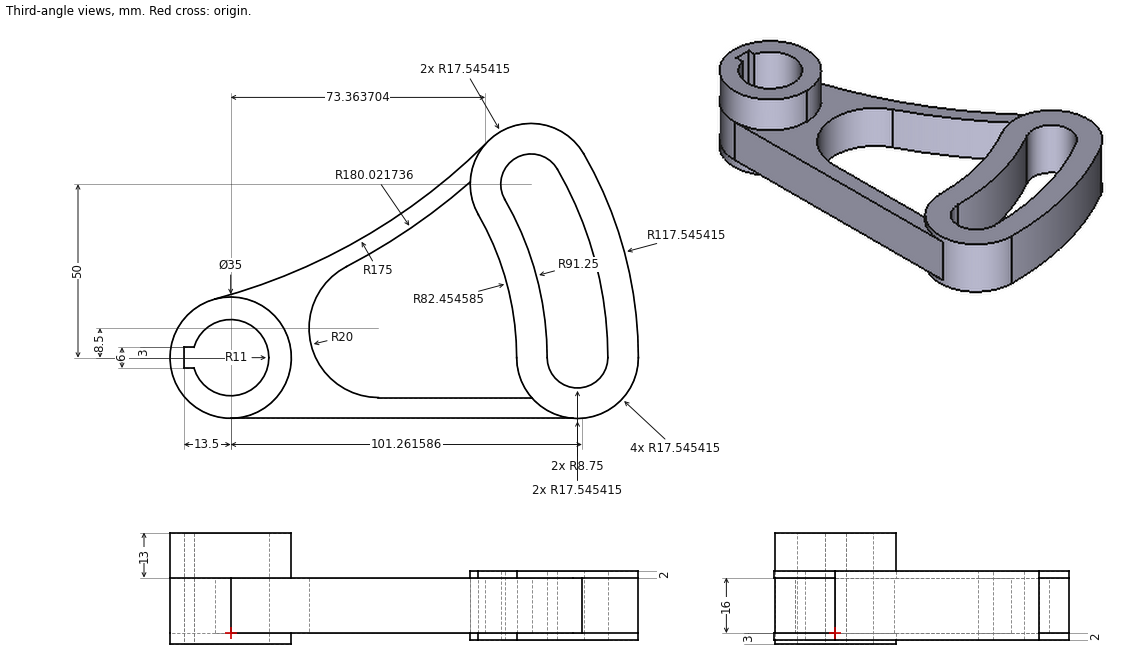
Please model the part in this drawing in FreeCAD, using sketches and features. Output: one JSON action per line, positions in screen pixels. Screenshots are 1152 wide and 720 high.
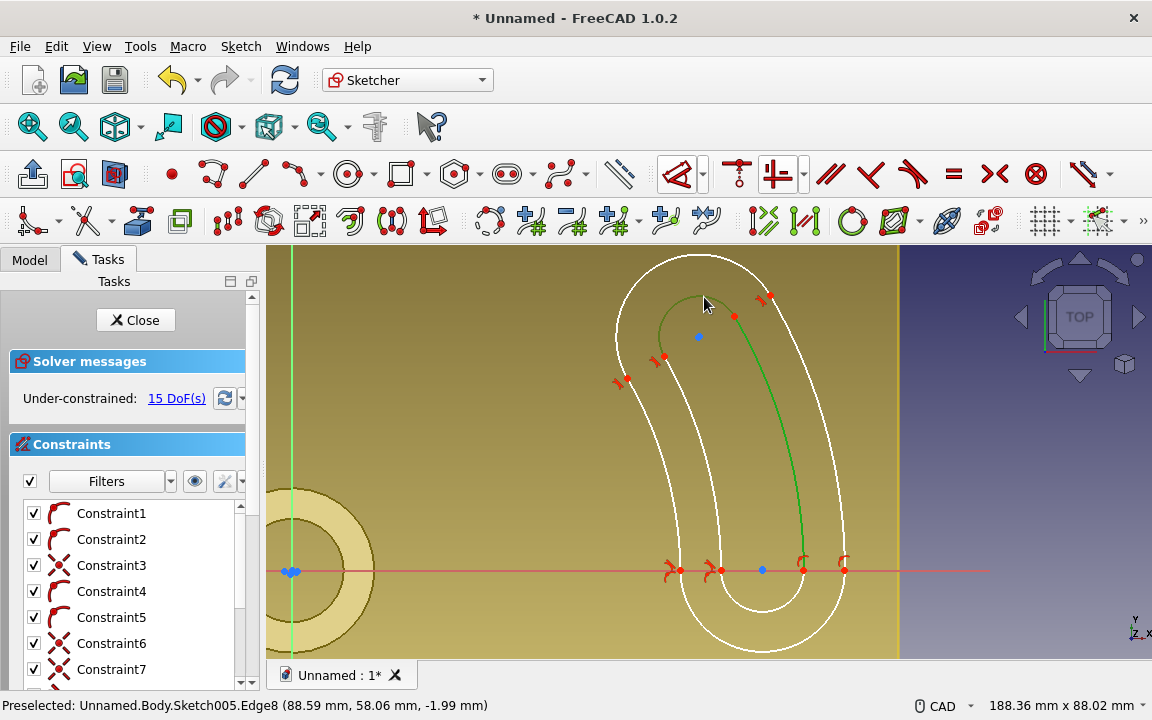
{"action": "left_click", "coordinate": [913, 174]}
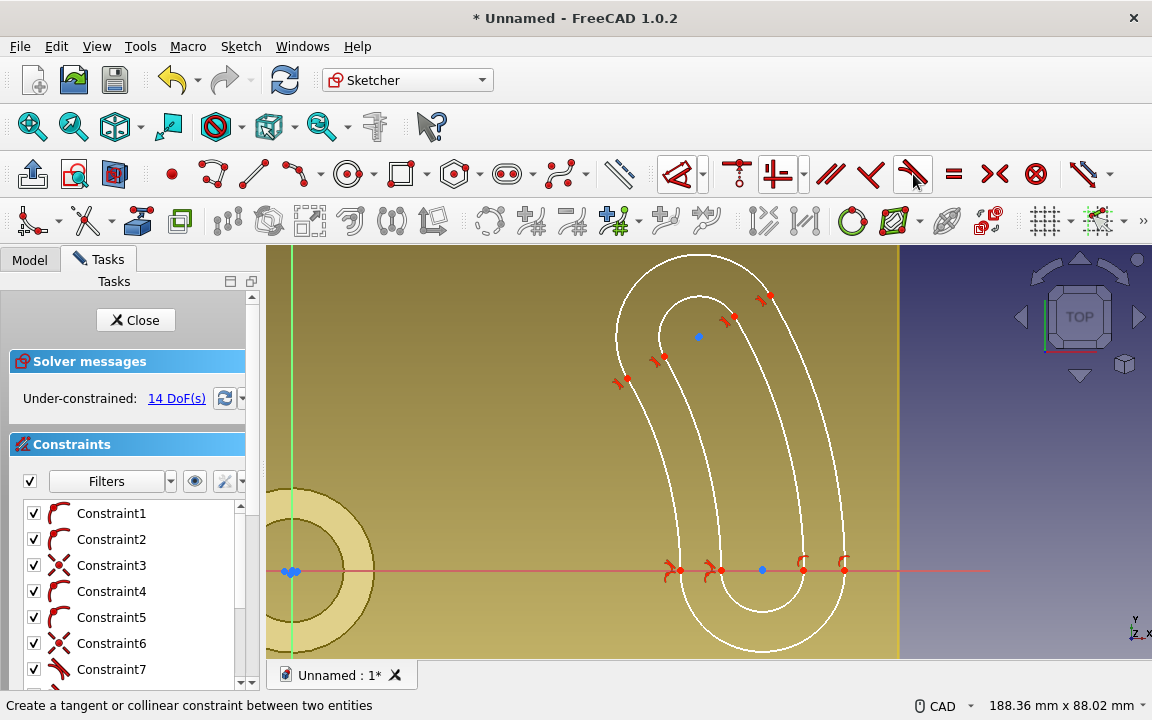
{"action": "left_click", "coordinate": [675, 510]}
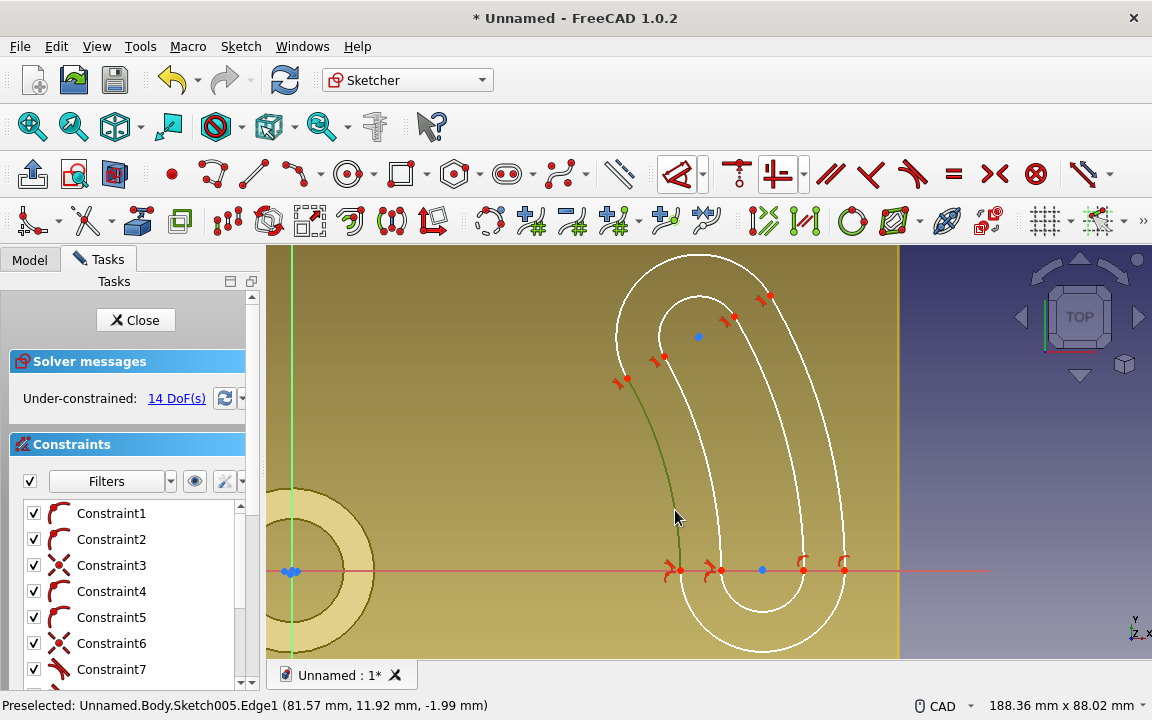
{"action": "left_click", "coordinate": [838, 484]}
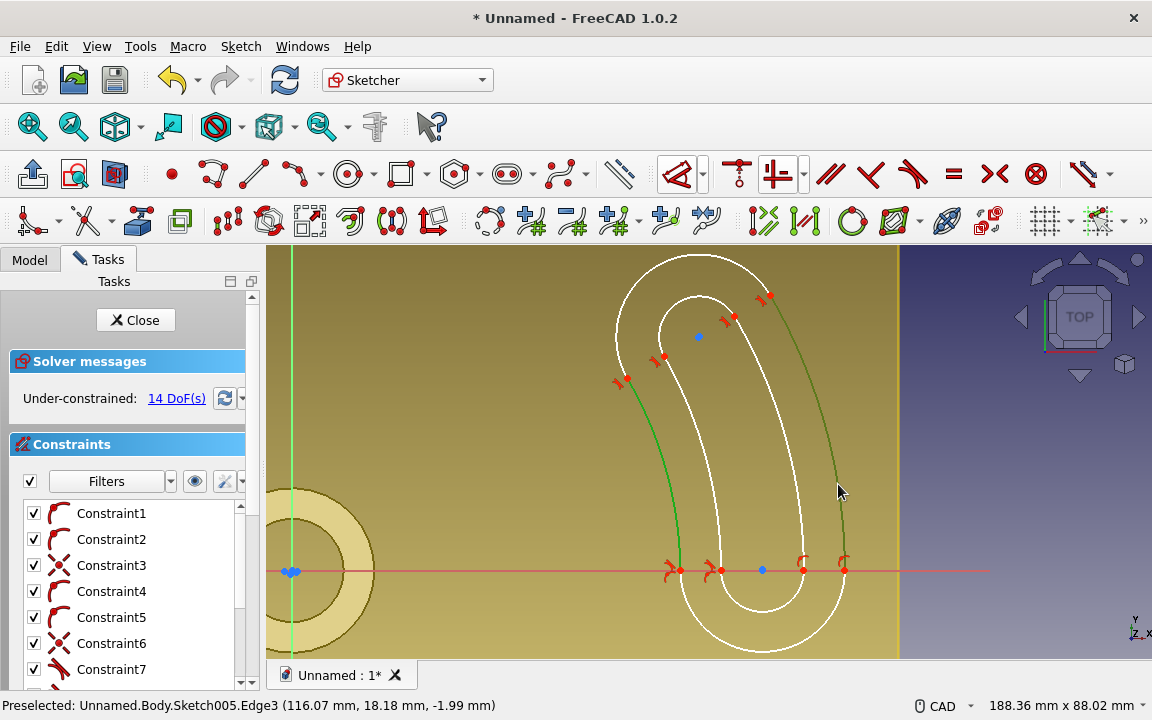
{"action": "left_click", "coordinate": [737, 174]}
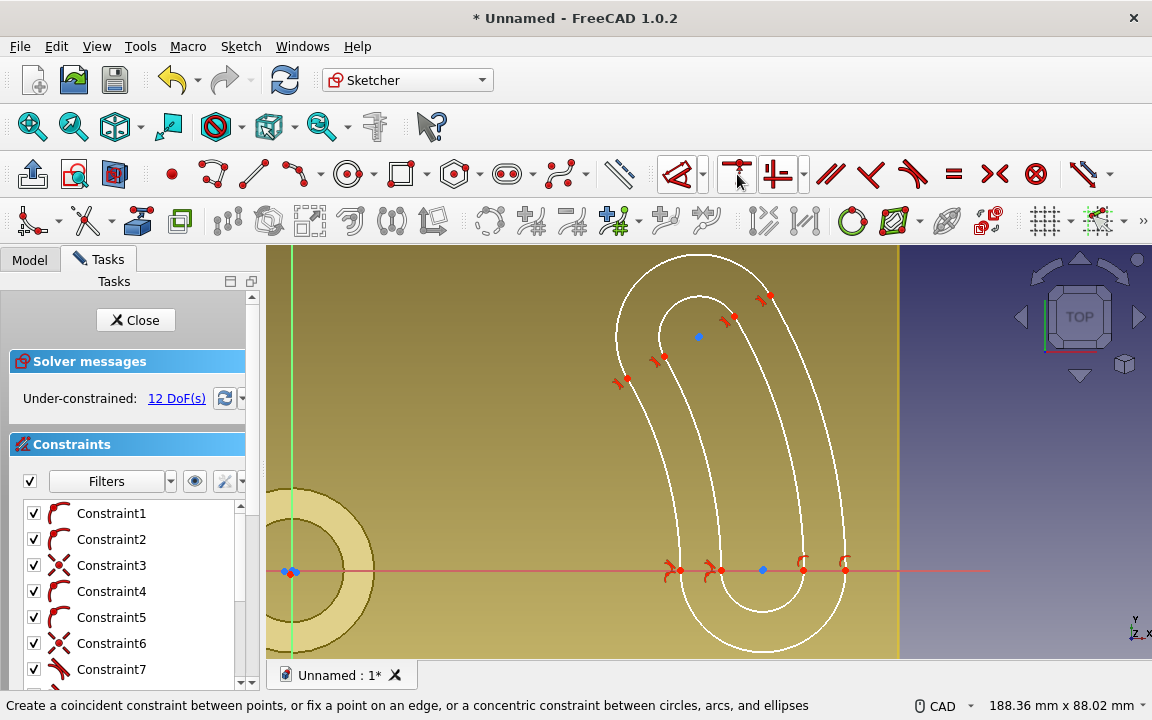
{"action": "left_click", "coordinate": [675, 510]}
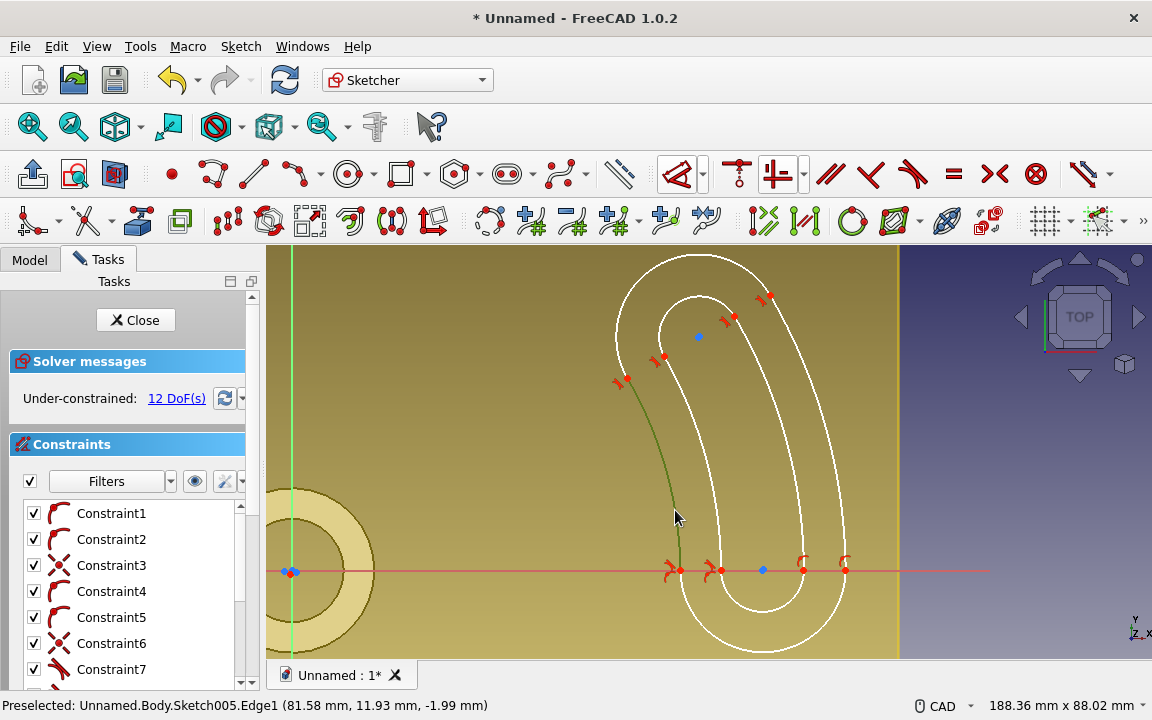
{"action": "left_click", "coordinate": [716, 504]}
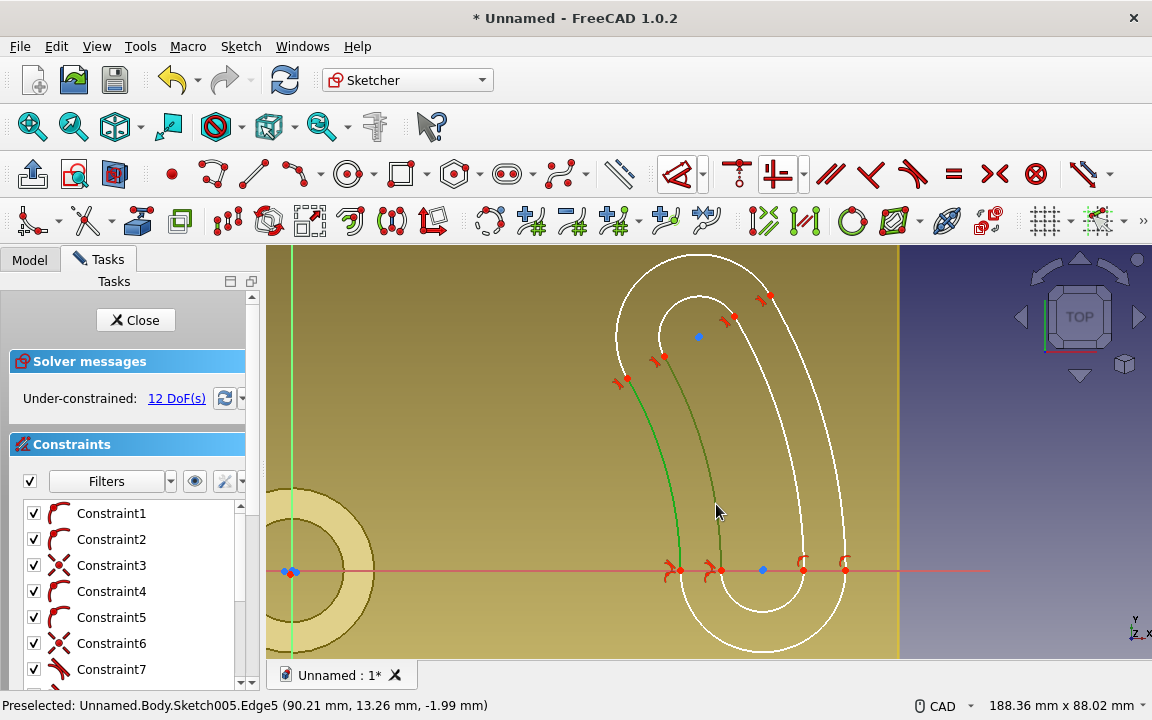
{"action": "left_click", "coordinate": [737, 174]}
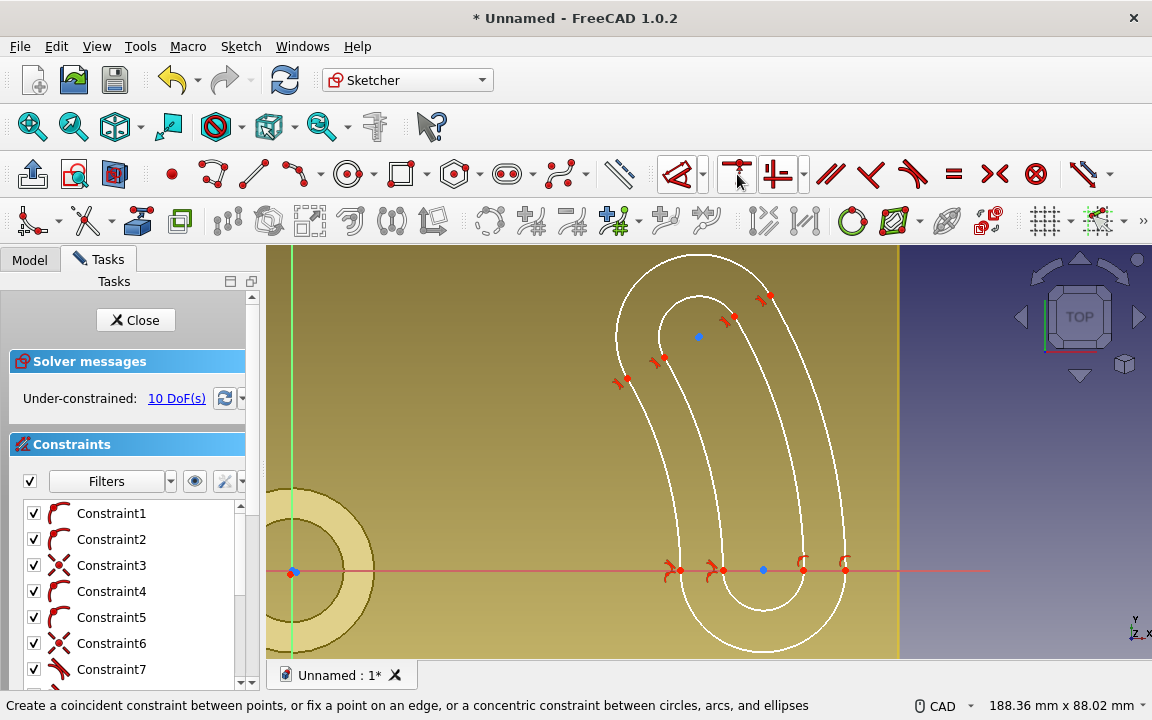
{"action": "left_click", "coordinate": [675, 510]}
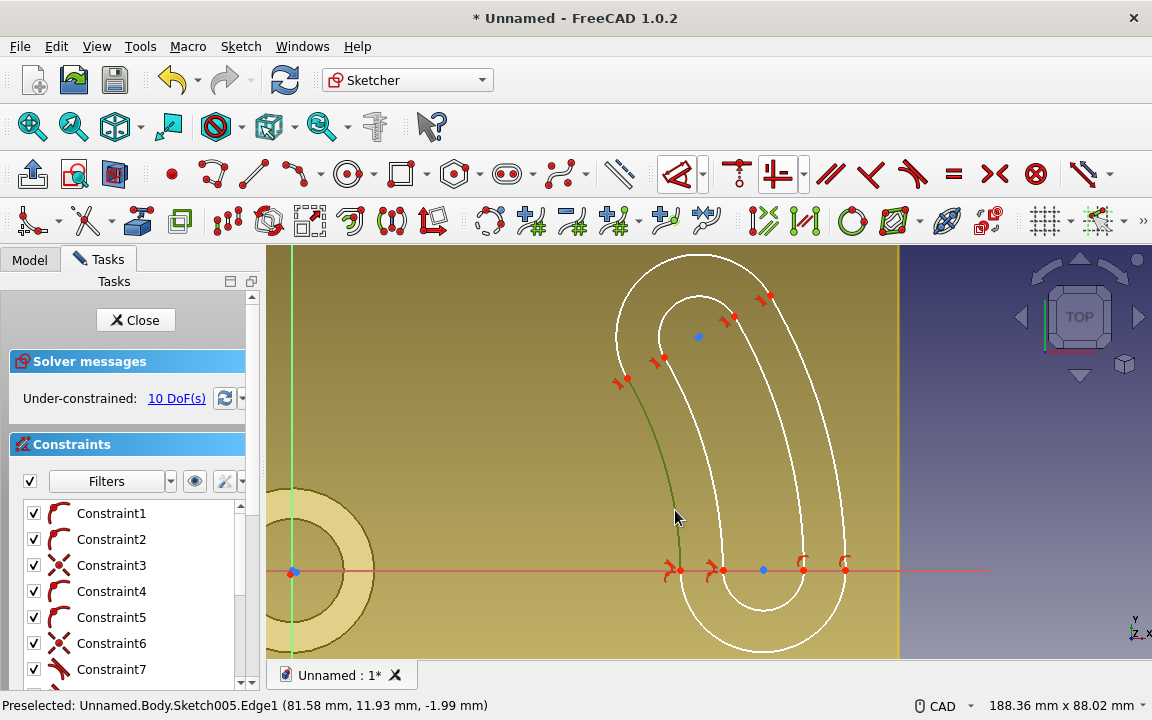
{"action": "left_click", "coordinate": [797, 491]}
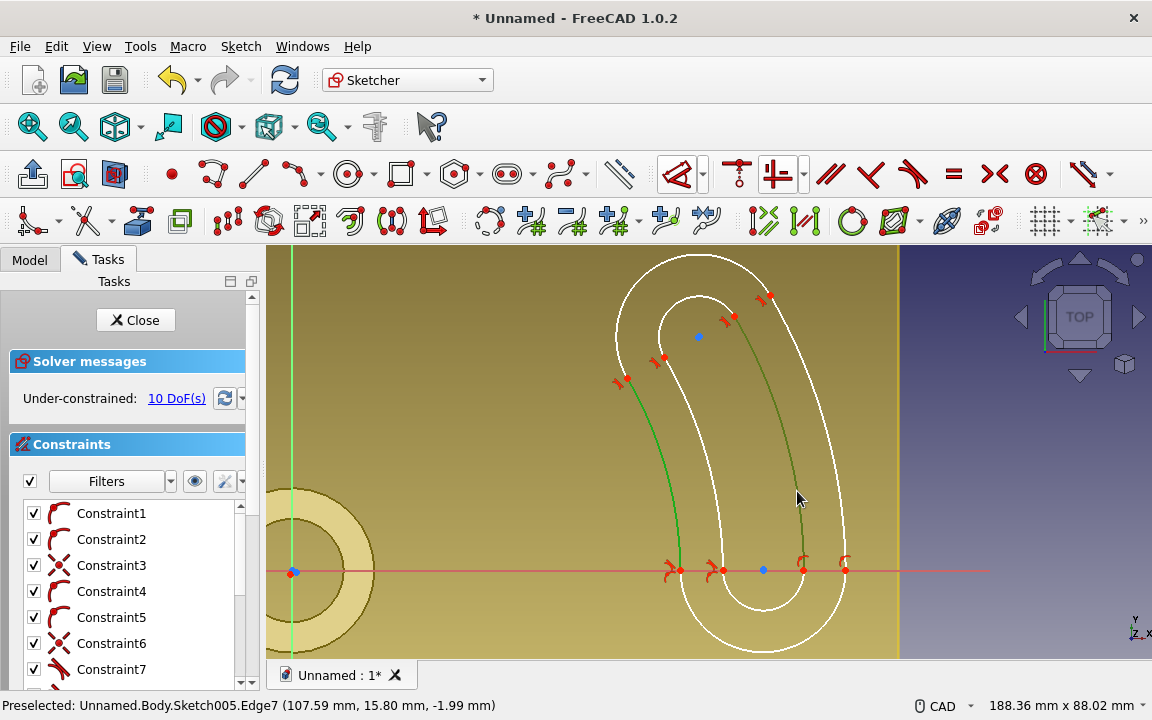
{"action": "left_click", "coordinate": [737, 174]}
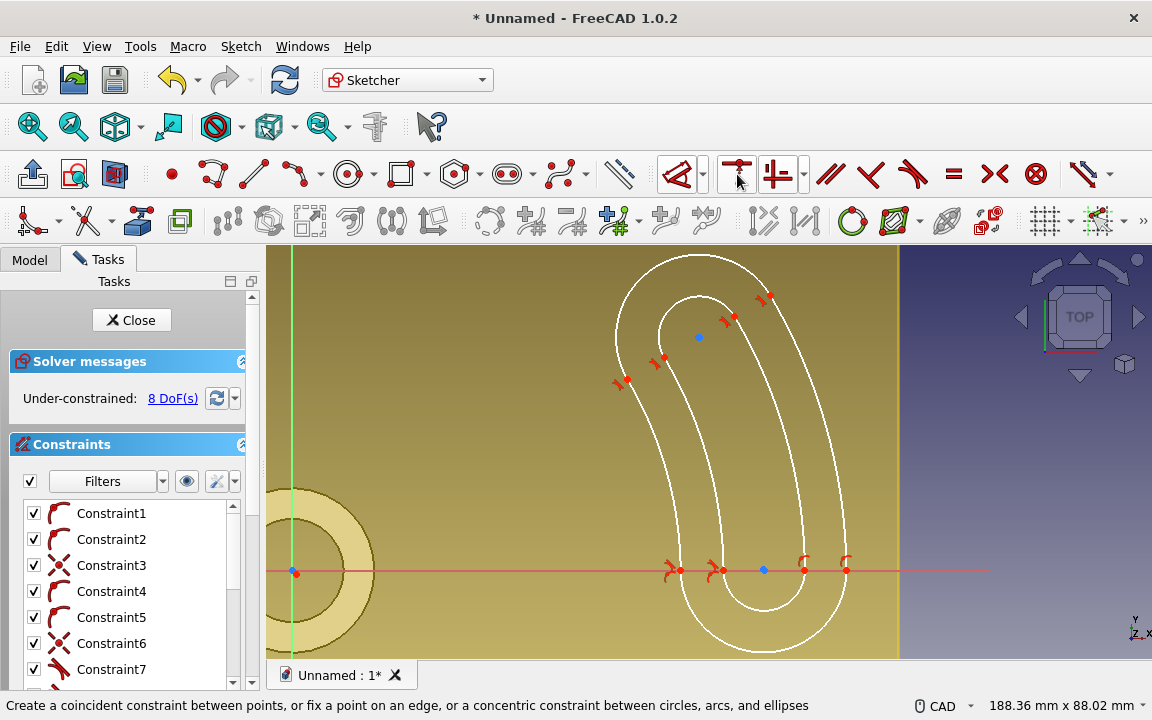
{"action": "left_click", "coordinate": [623, 305]}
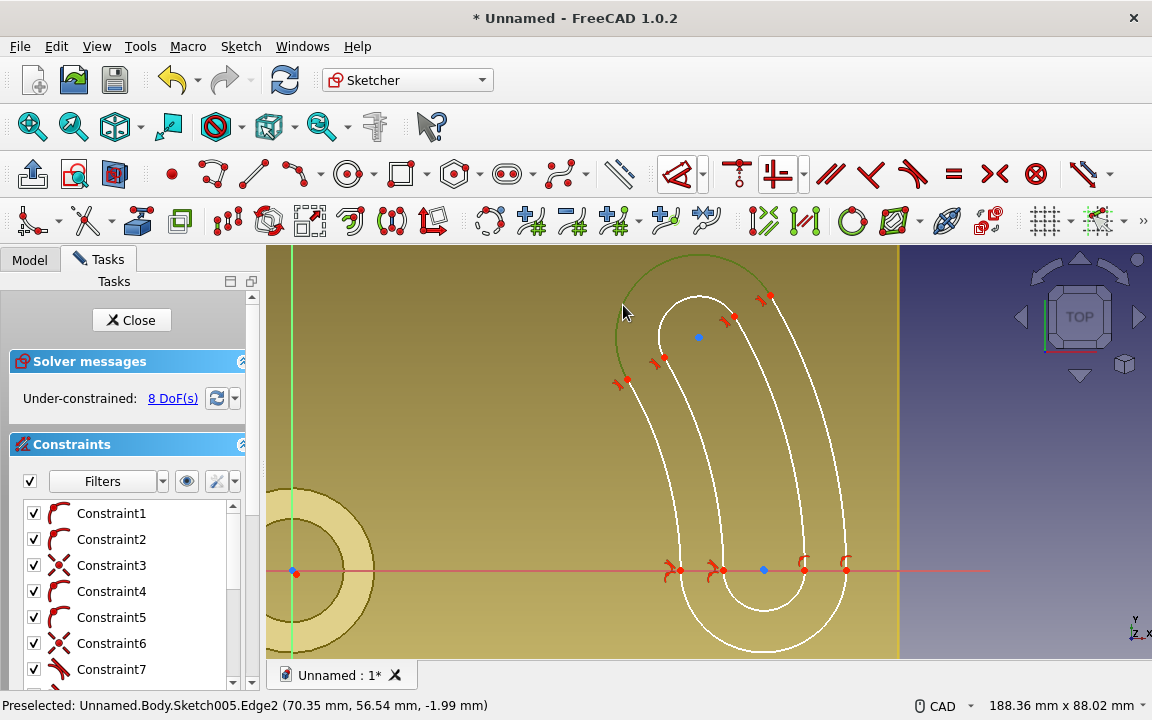
{"action": "left_click", "coordinate": [703, 297]}